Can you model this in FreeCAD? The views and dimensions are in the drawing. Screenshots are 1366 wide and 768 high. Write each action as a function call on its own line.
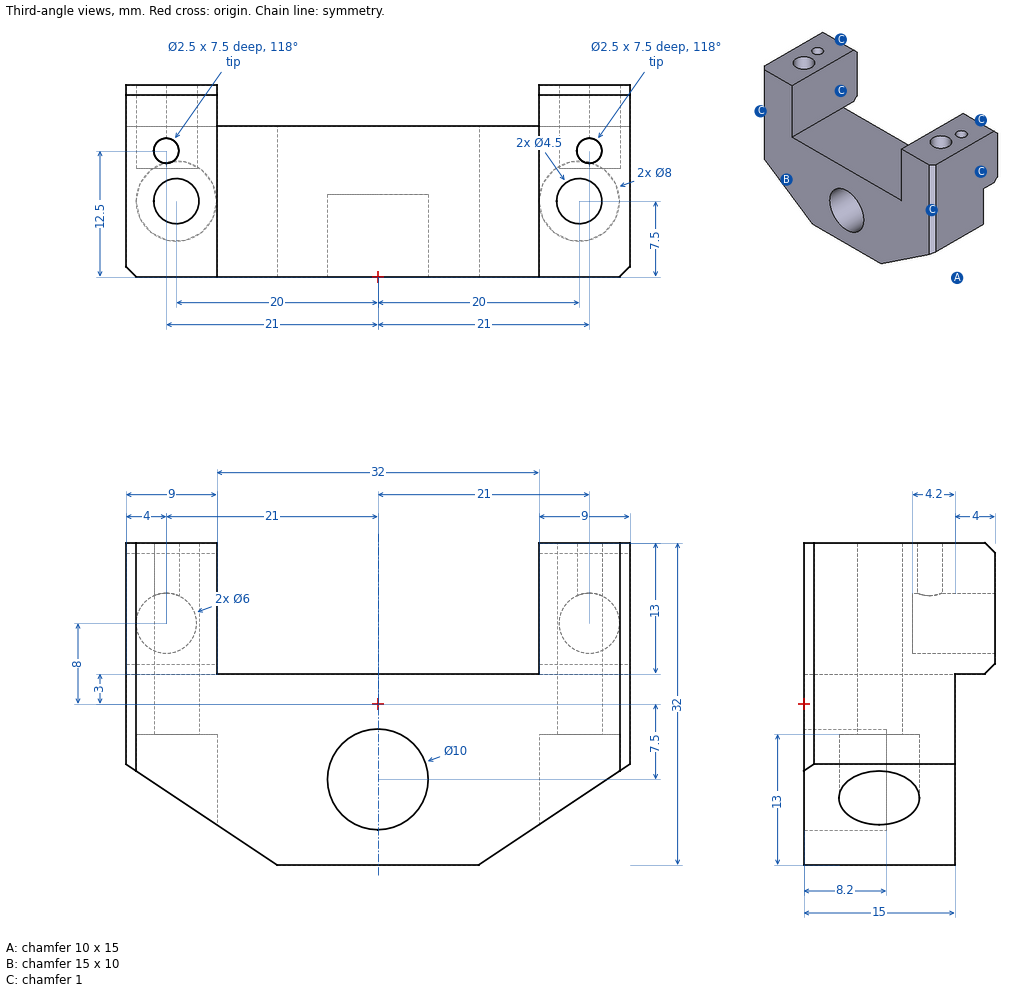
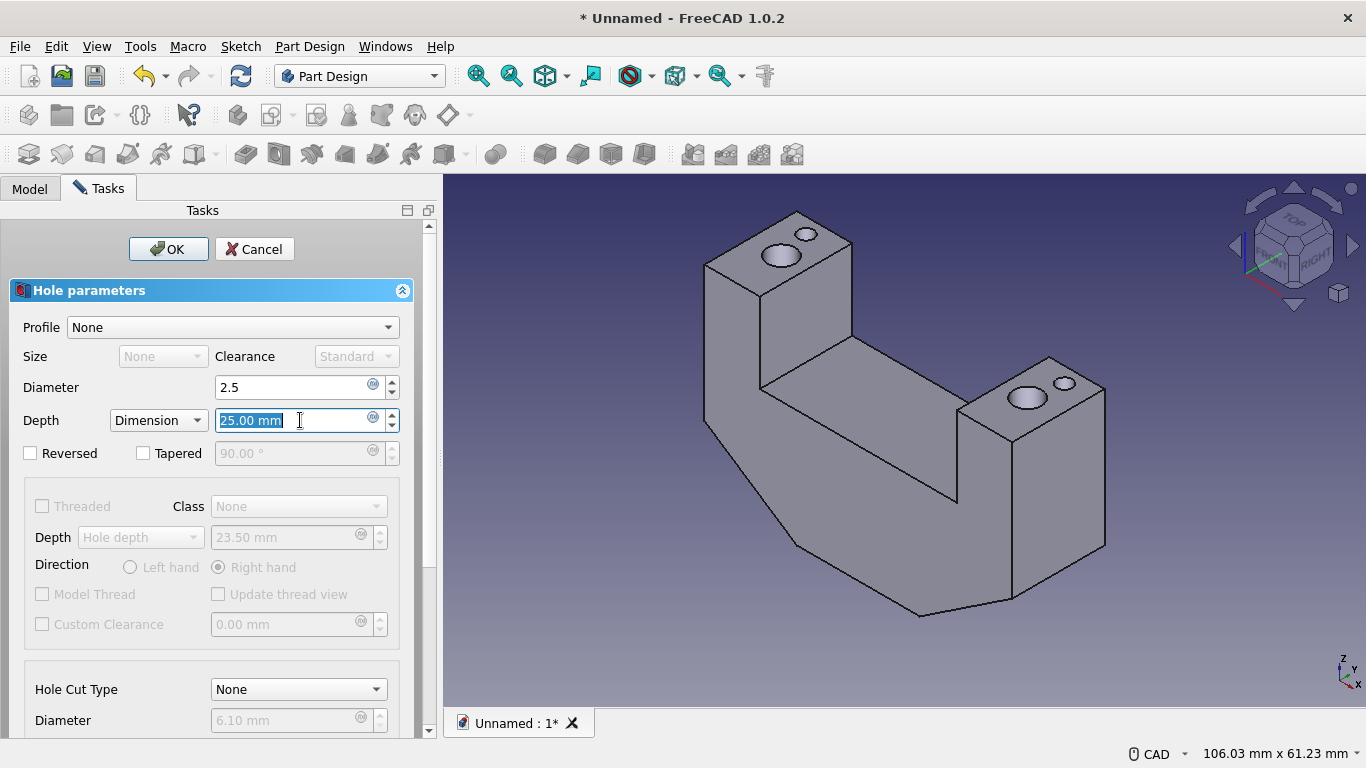
text(7.5)
key(Tab)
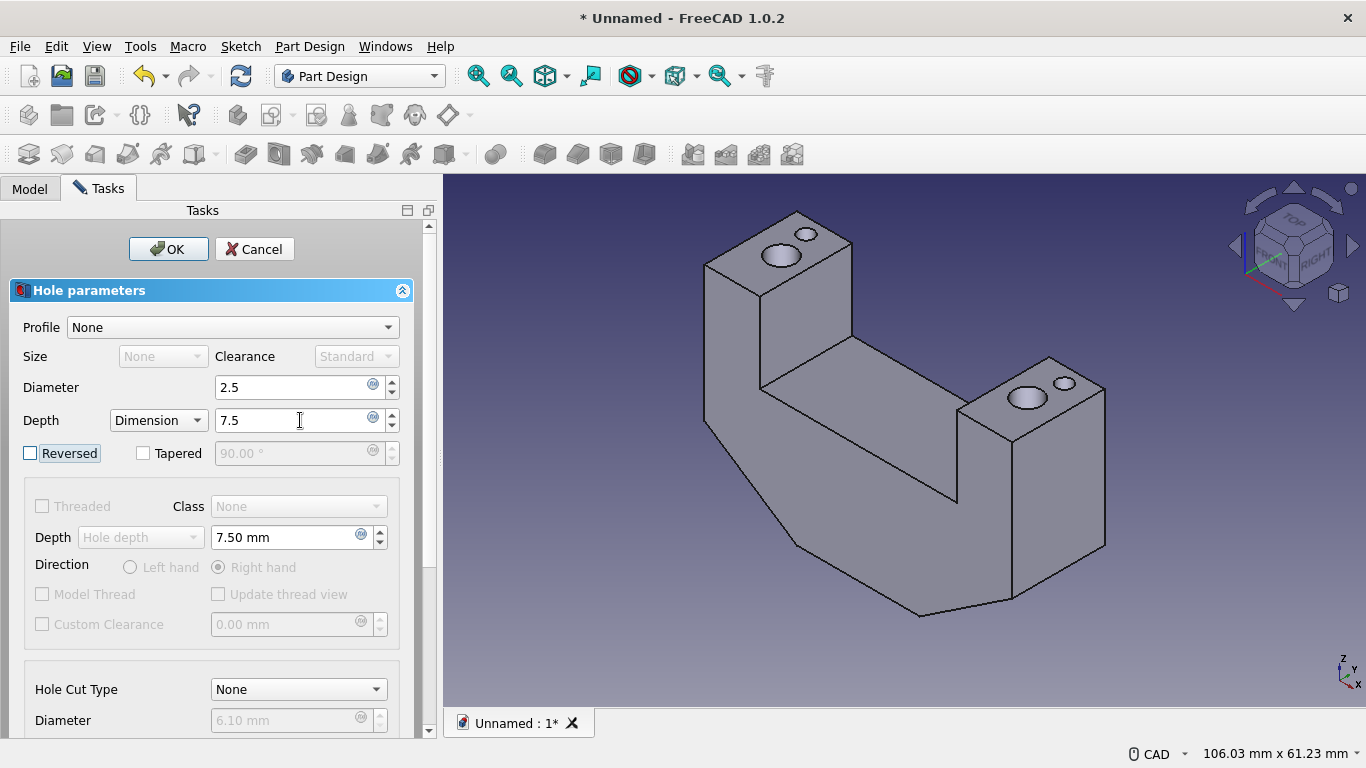
click(169, 249)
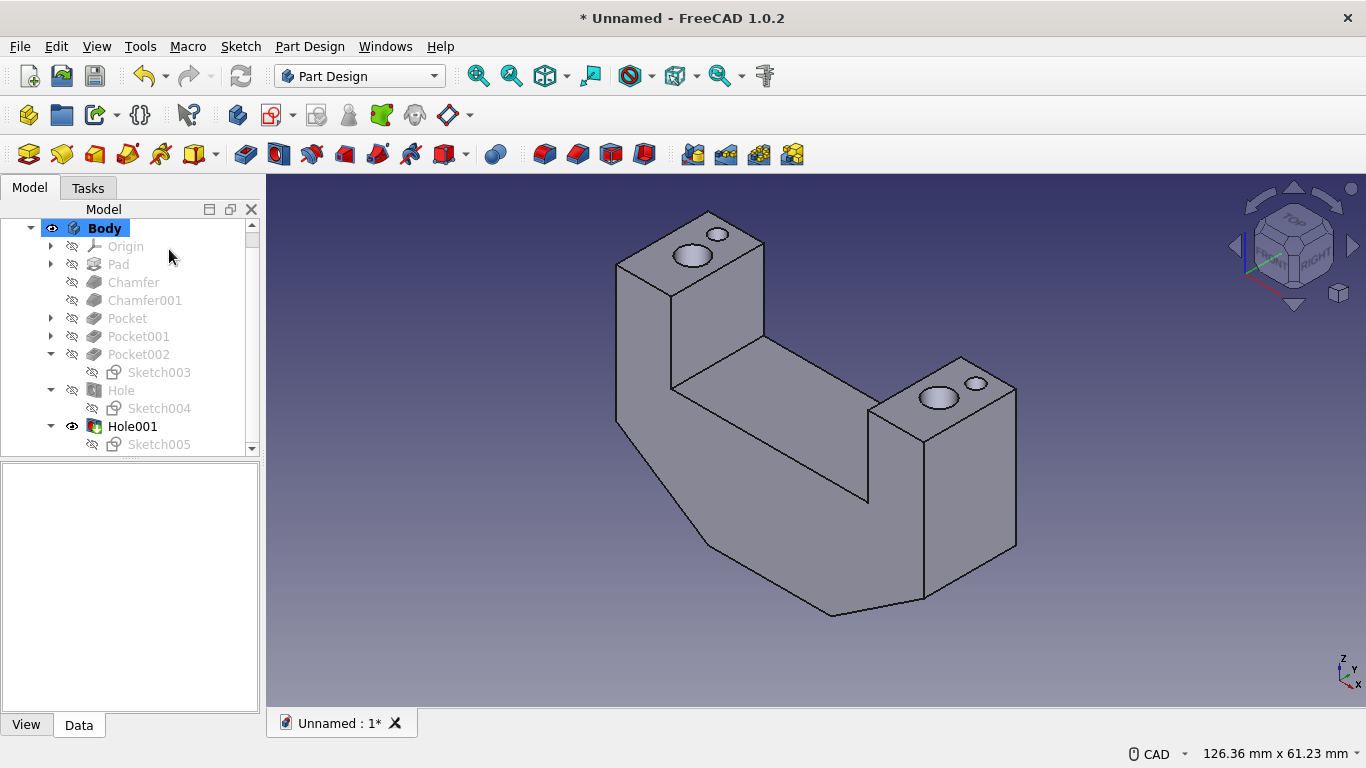
click(51, 246)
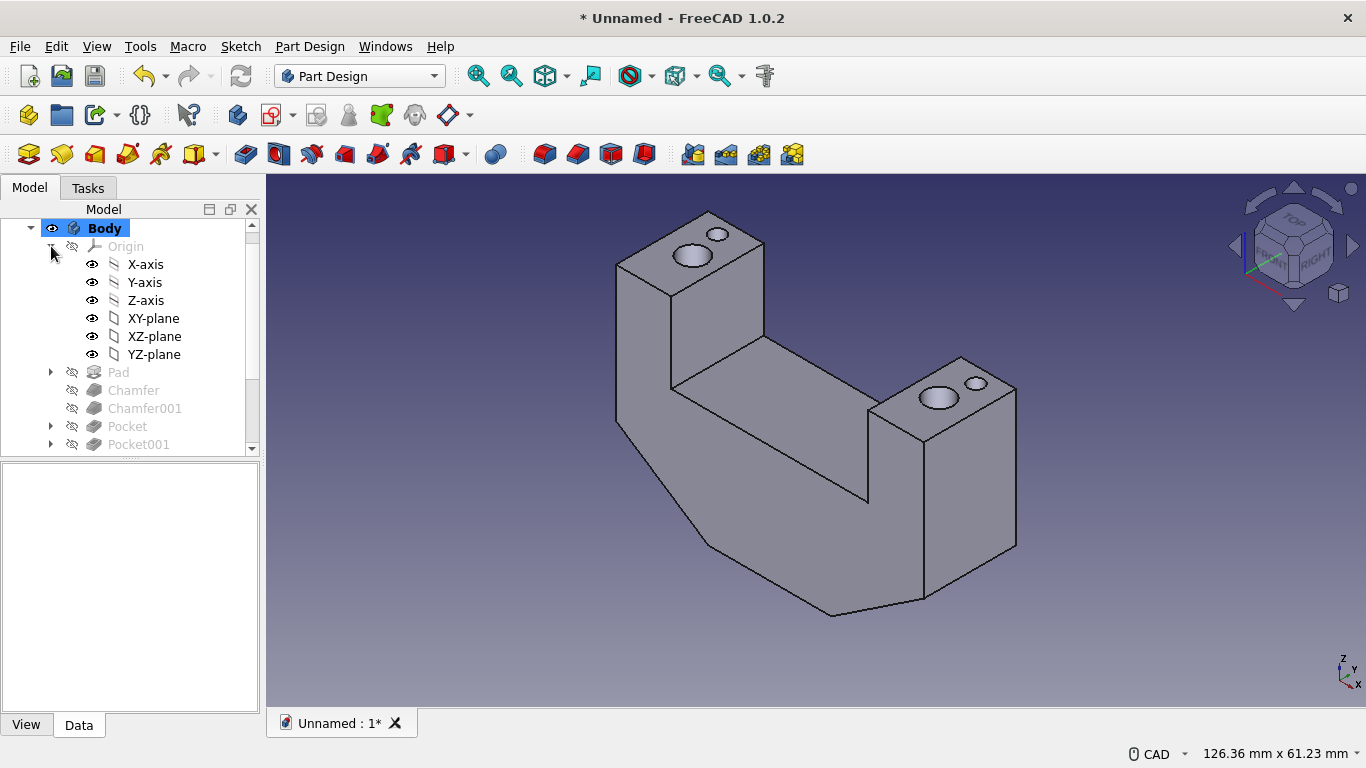
click(137, 336)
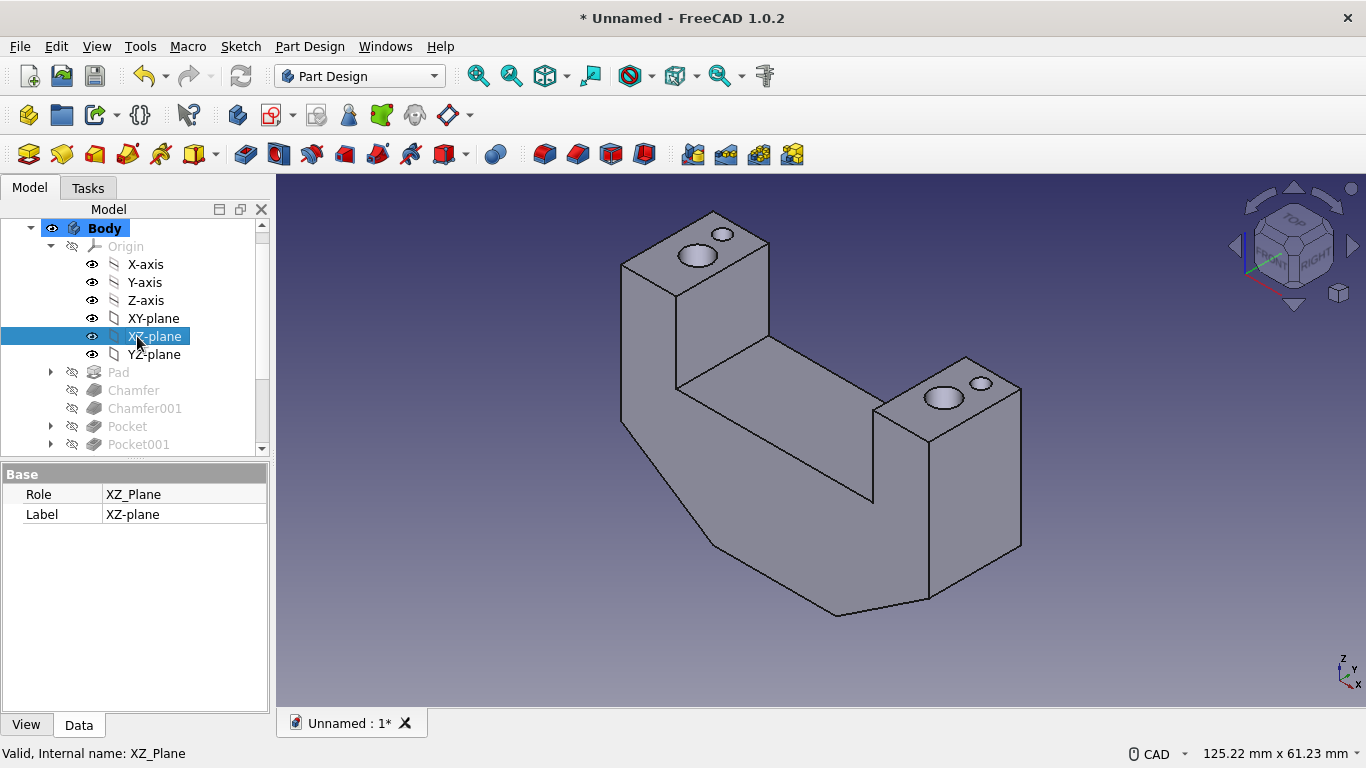
click(448, 116)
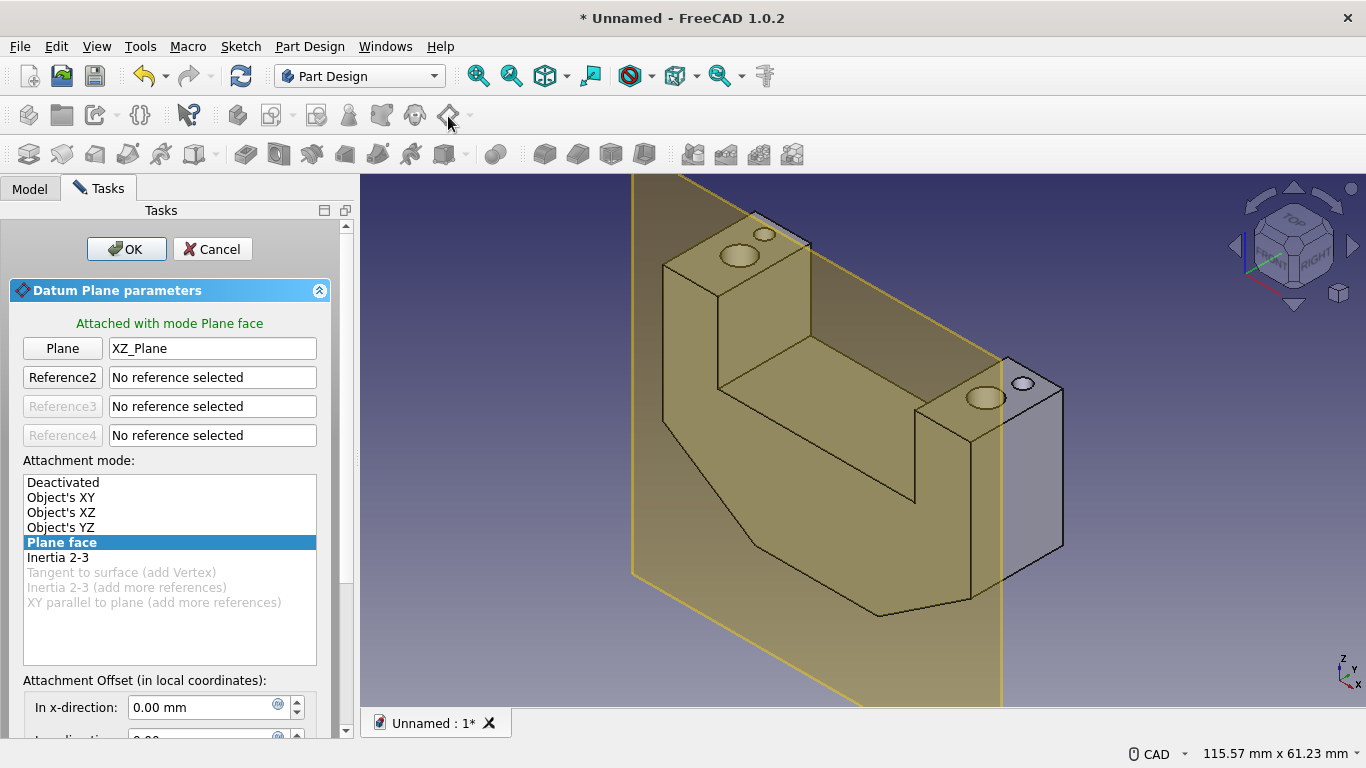
scroll(346, 479, down, 2)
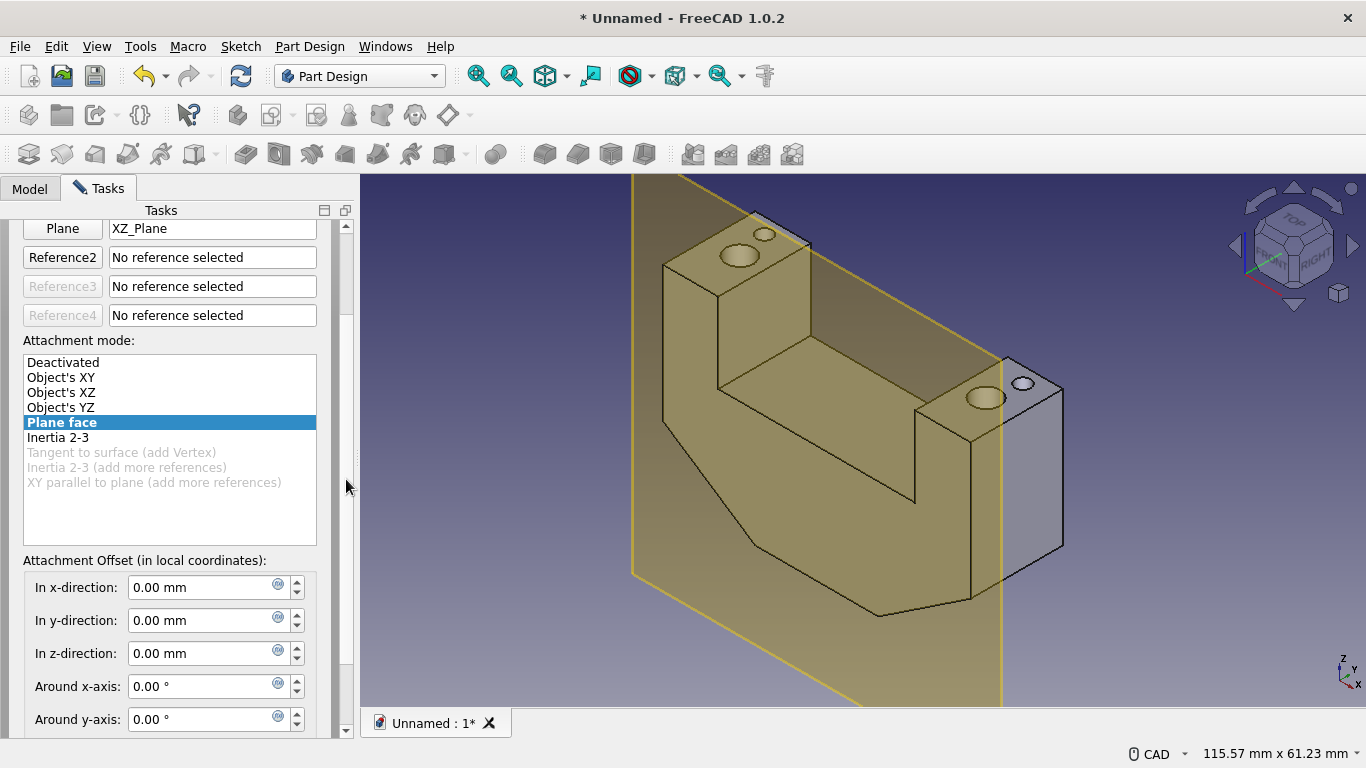
triple_click(210, 654)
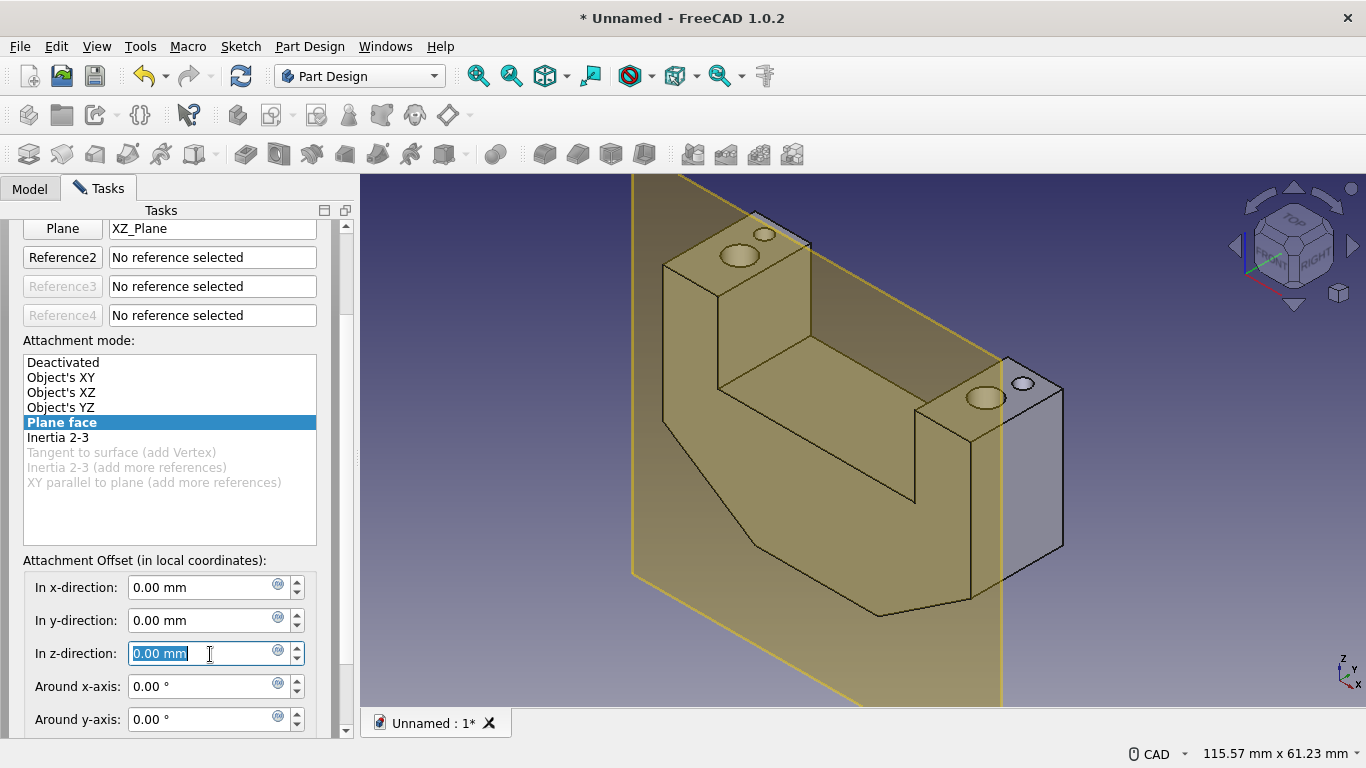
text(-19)
key(Tab)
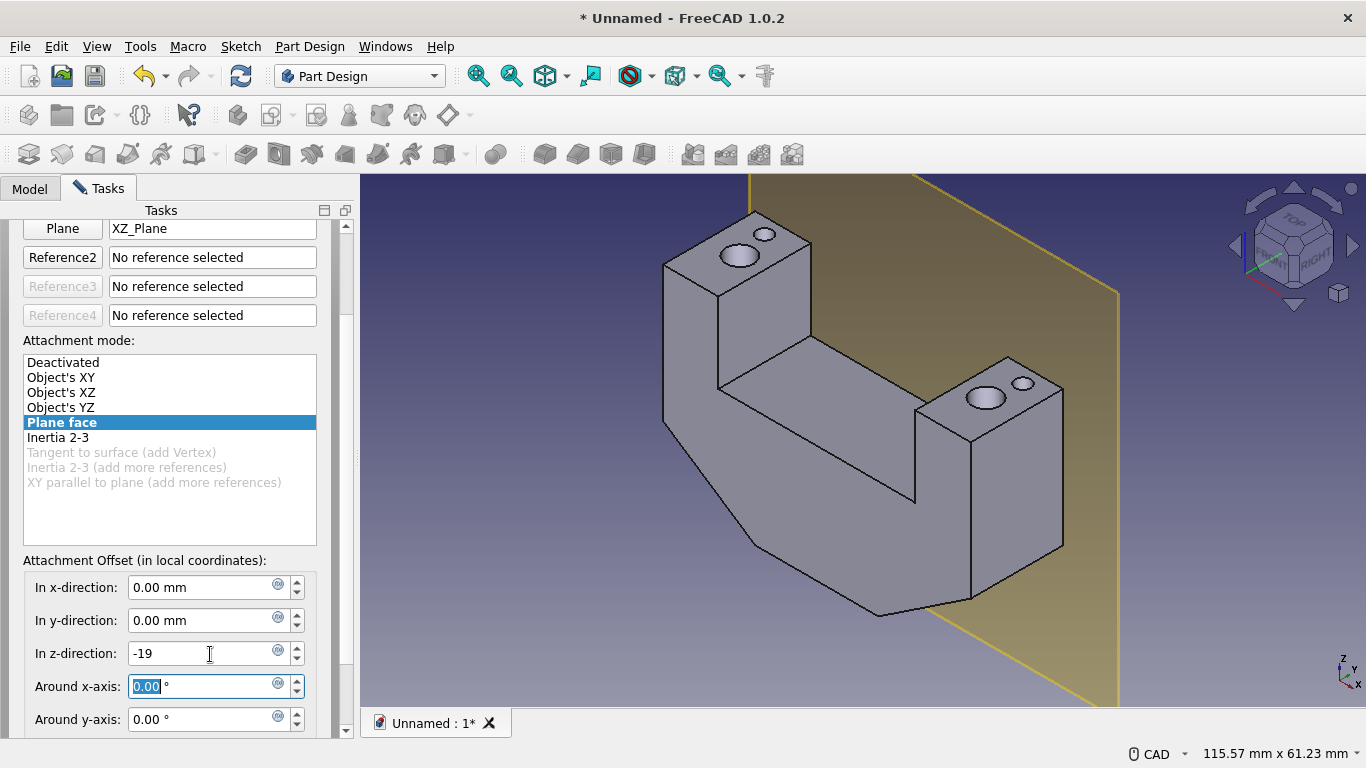
scroll(346, 479, up, 3)